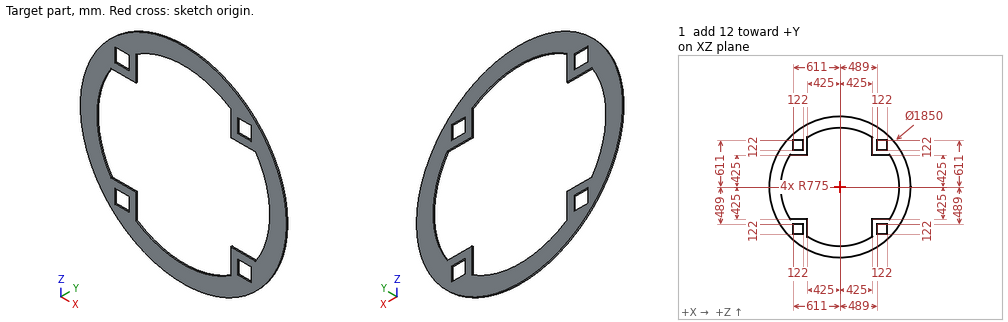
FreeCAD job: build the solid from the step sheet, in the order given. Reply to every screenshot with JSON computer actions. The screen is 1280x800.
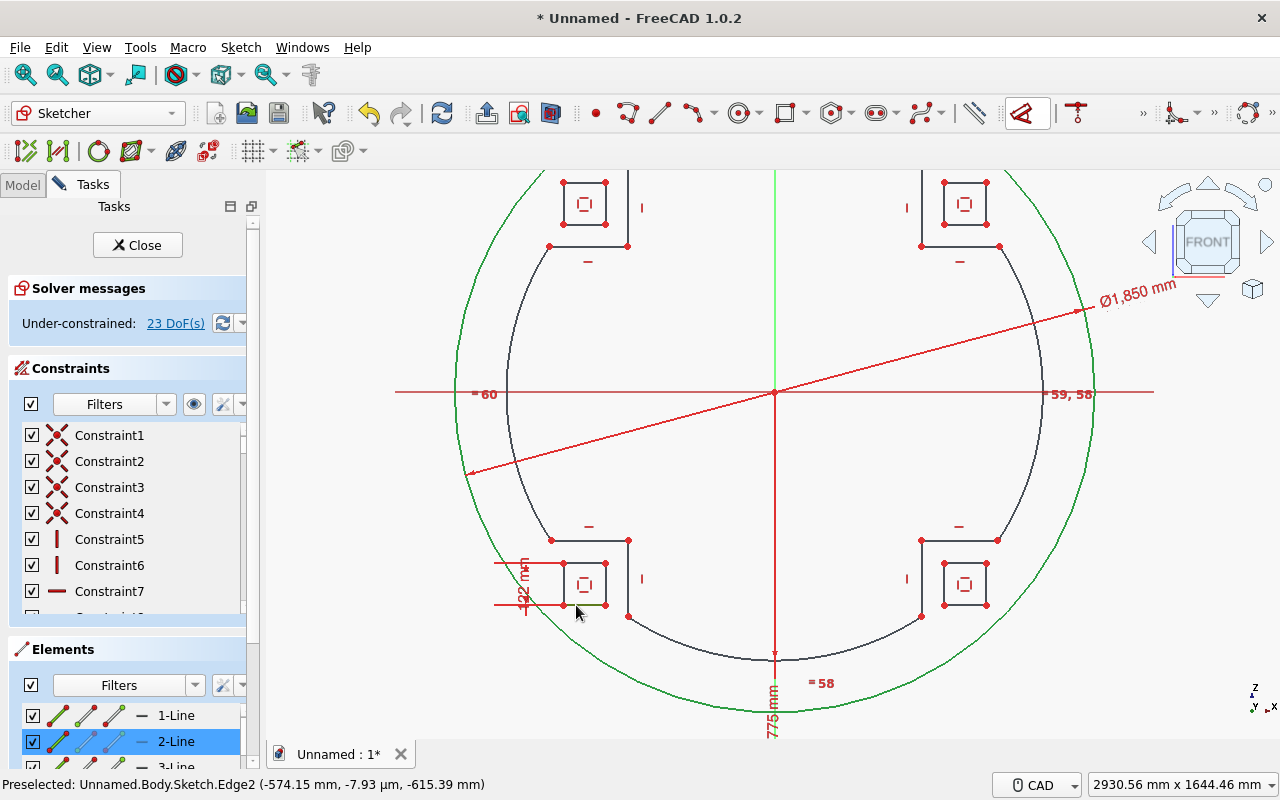
{"action": "key", "text": "l"}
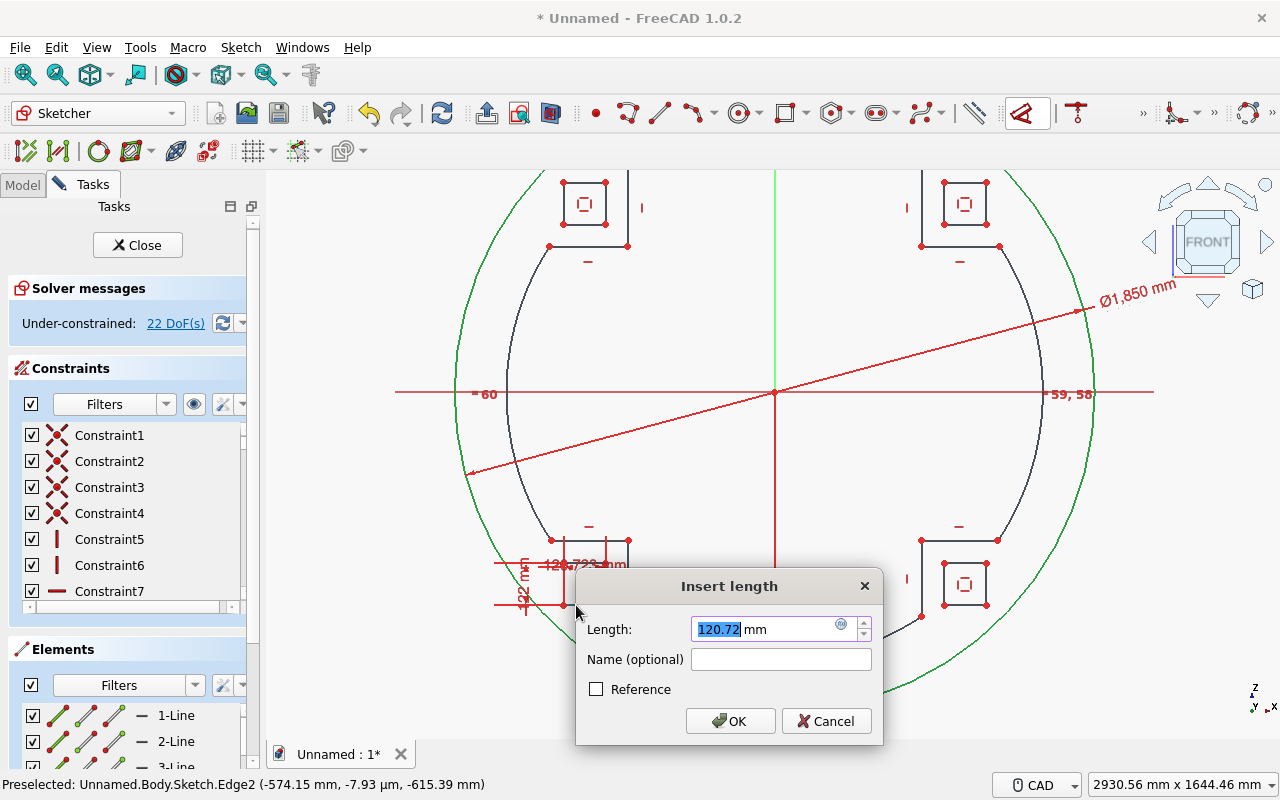
{"action": "type", "text": "122"}
{"action": "key", "text": "Return"}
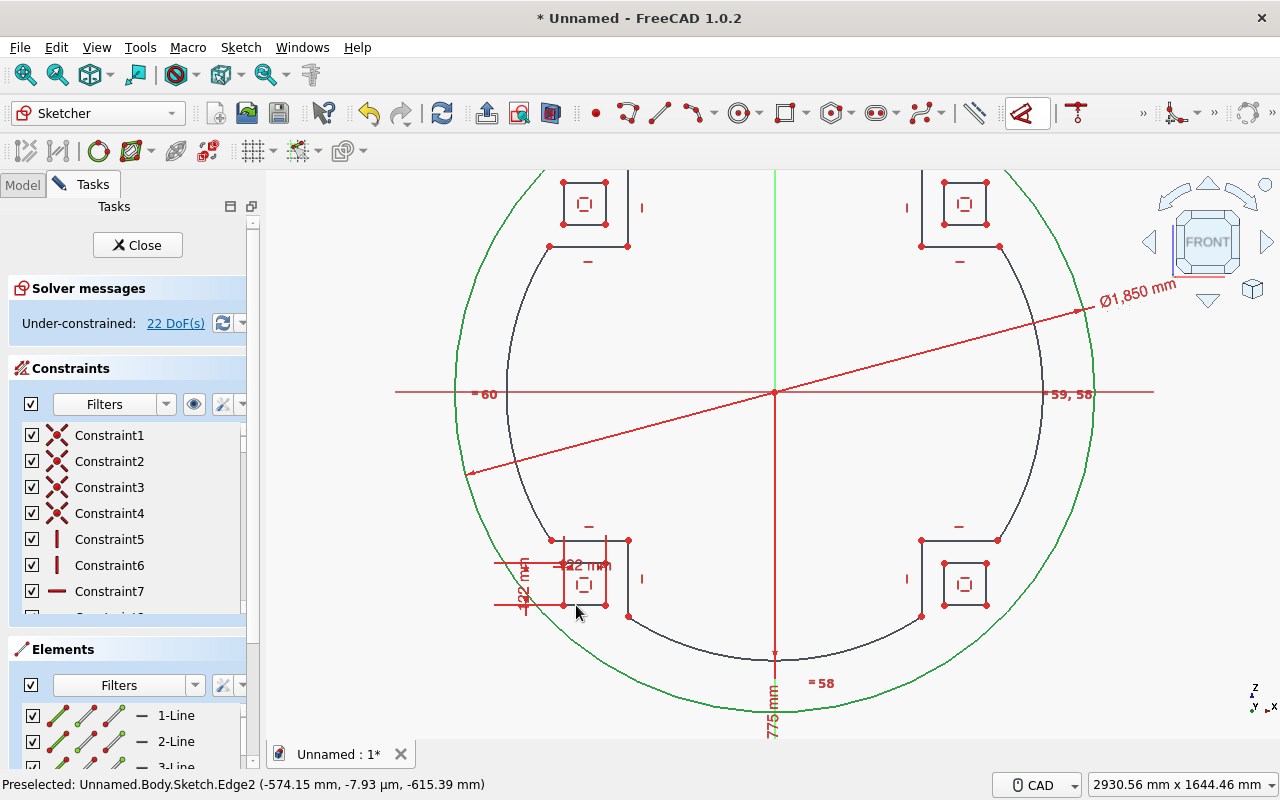
{"action": "left_click", "coordinate": [564, 212]}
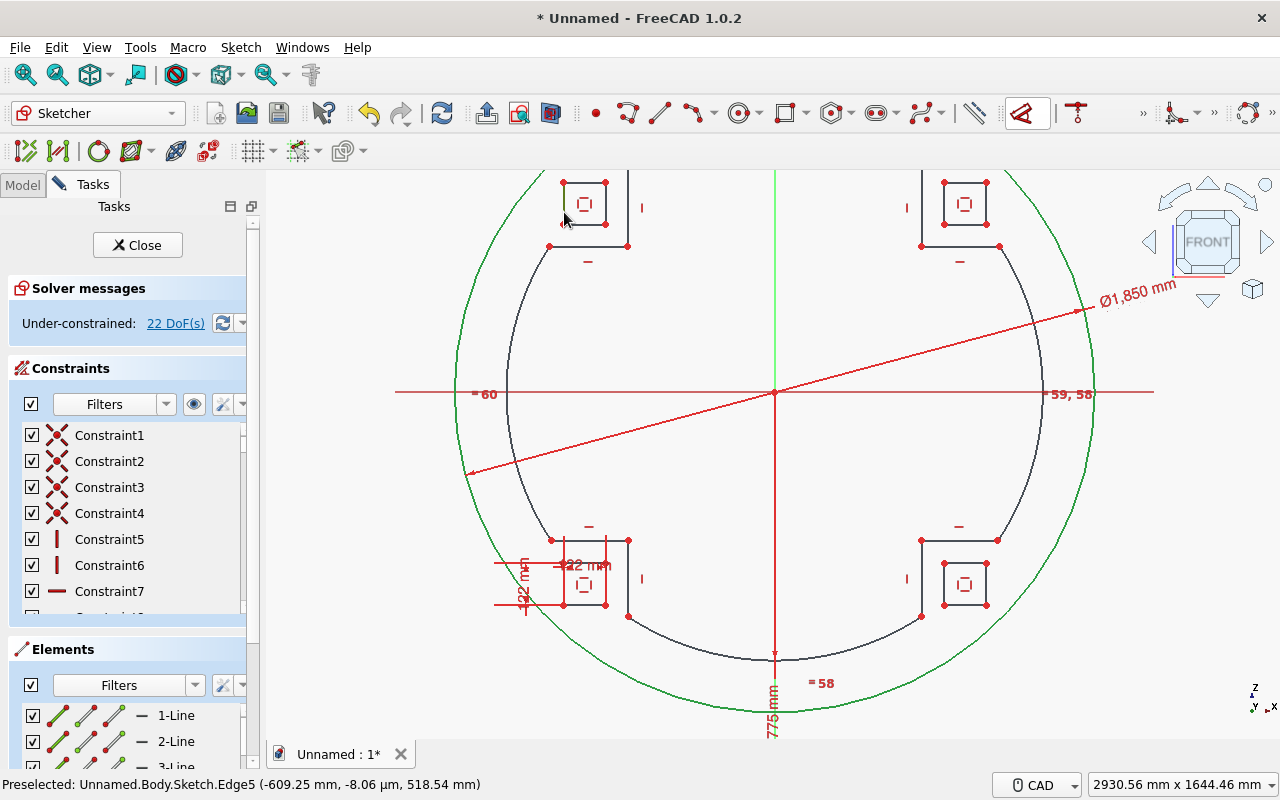
{"action": "key", "text": "i"}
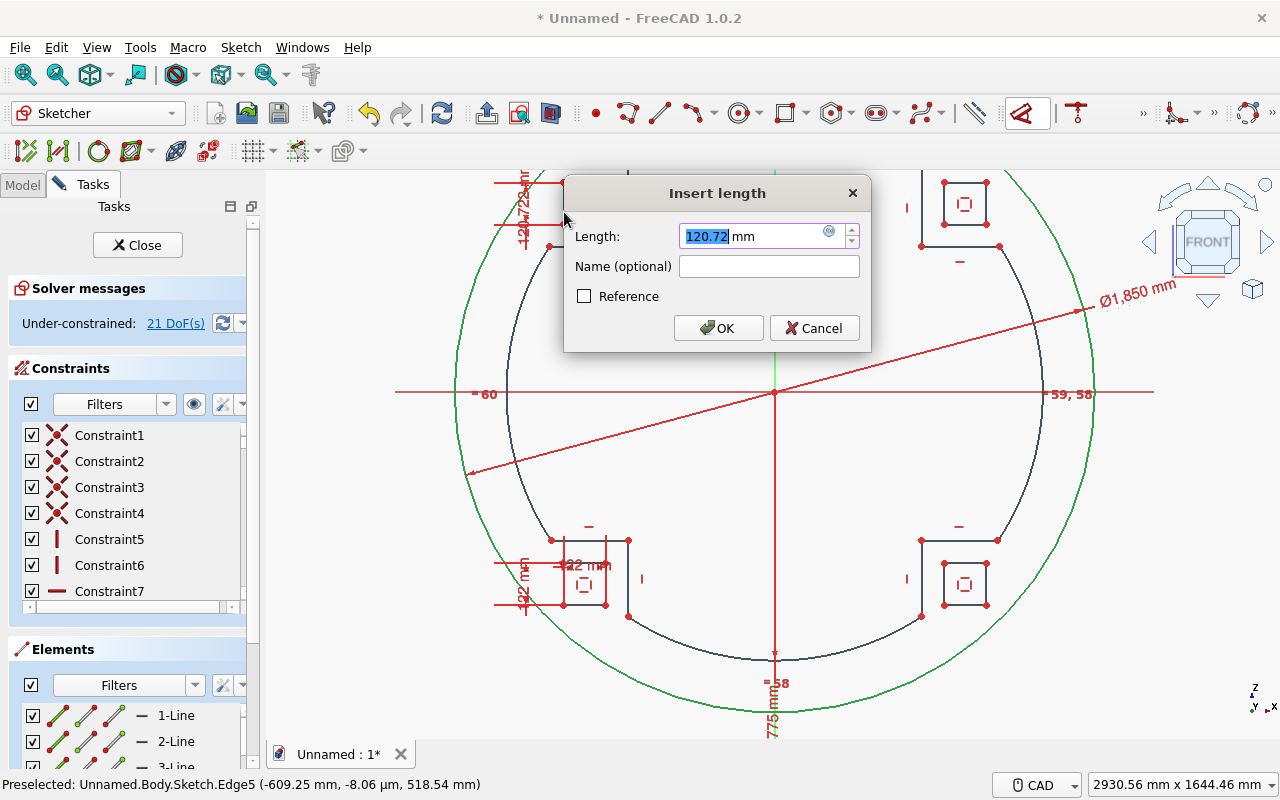
{"action": "type", "text": "122"}
{"action": "key", "text": "Return"}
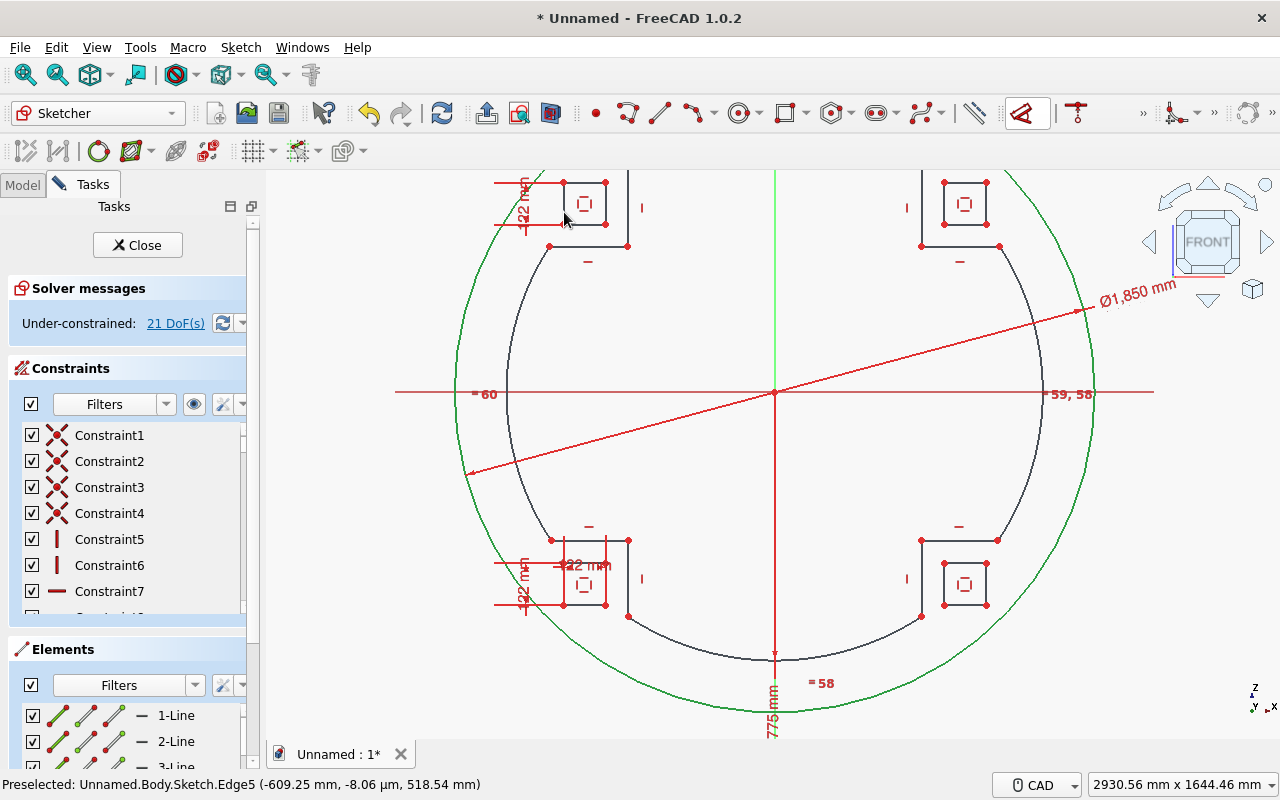
{"action": "left_click", "coordinate": [576, 225]}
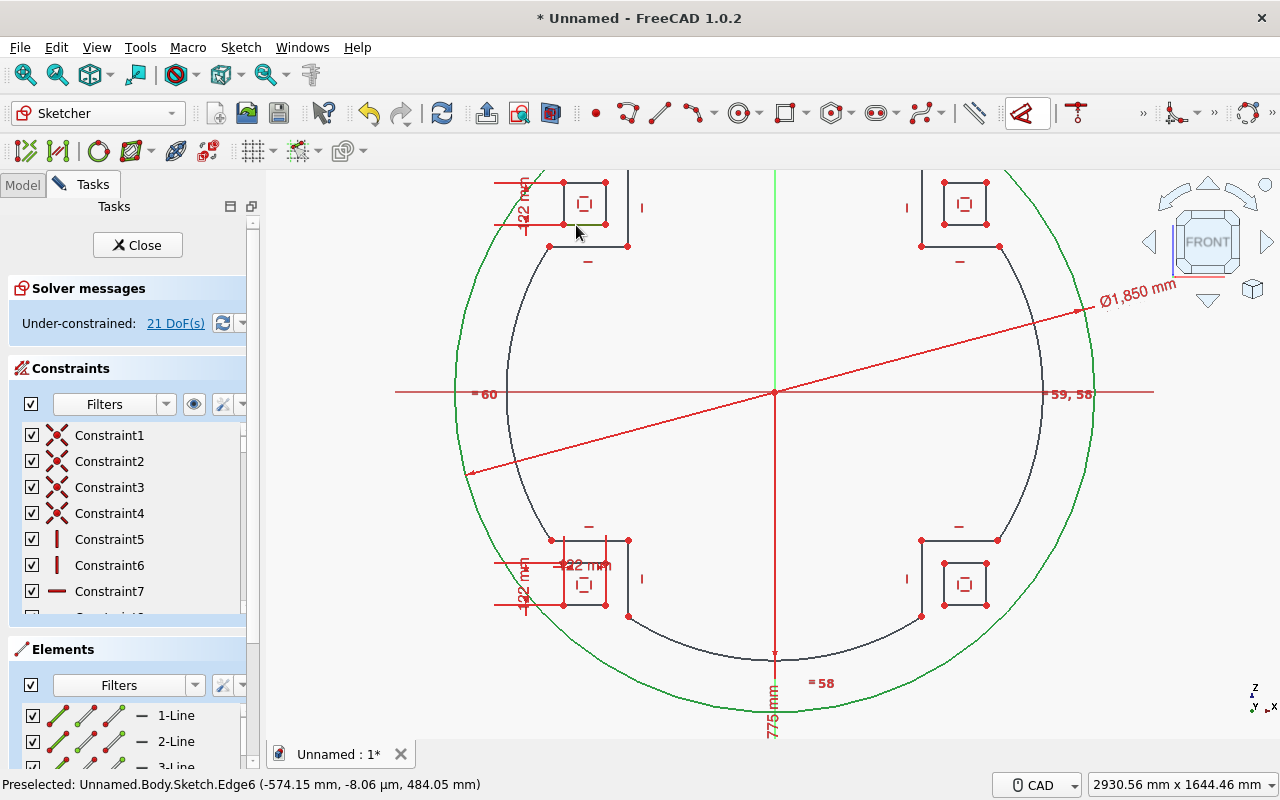
{"action": "key", "text": "l"}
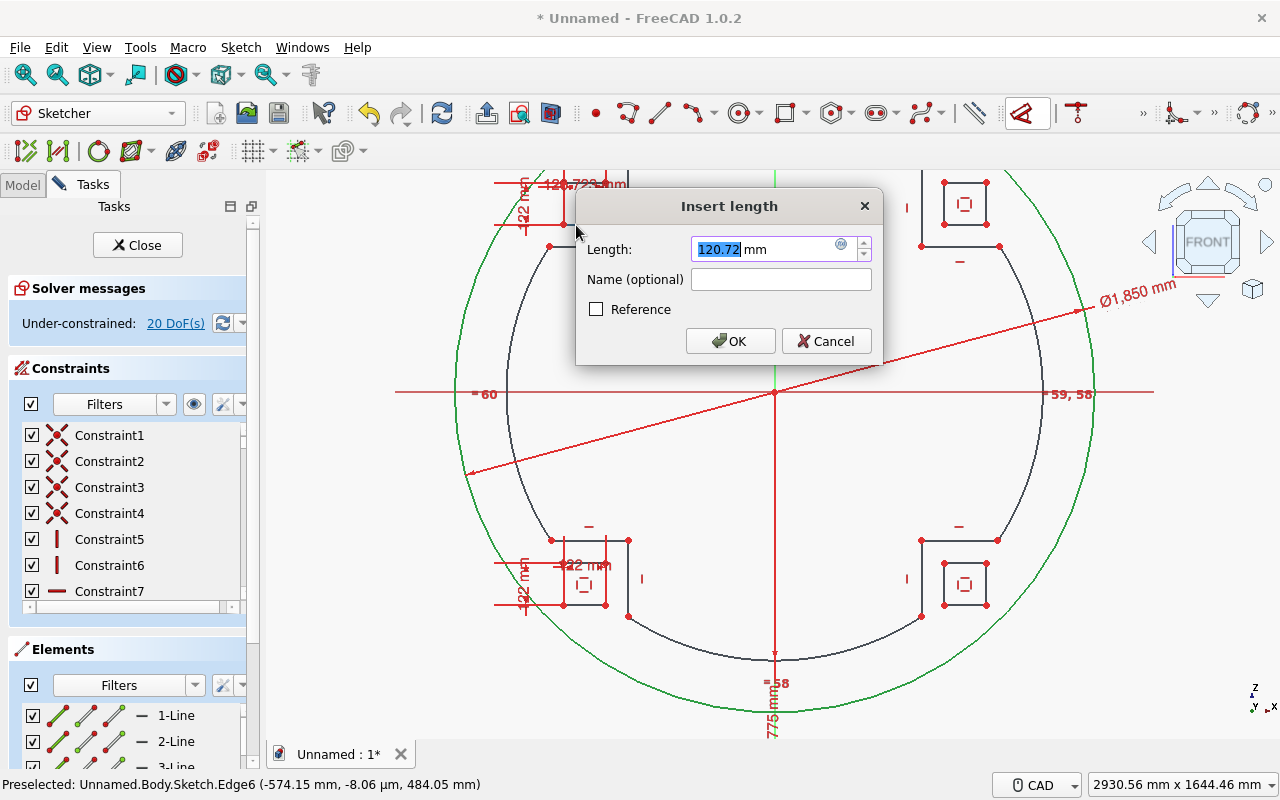
{"action": "type", "text": "122"}
{"action": "key", "text": "Return"}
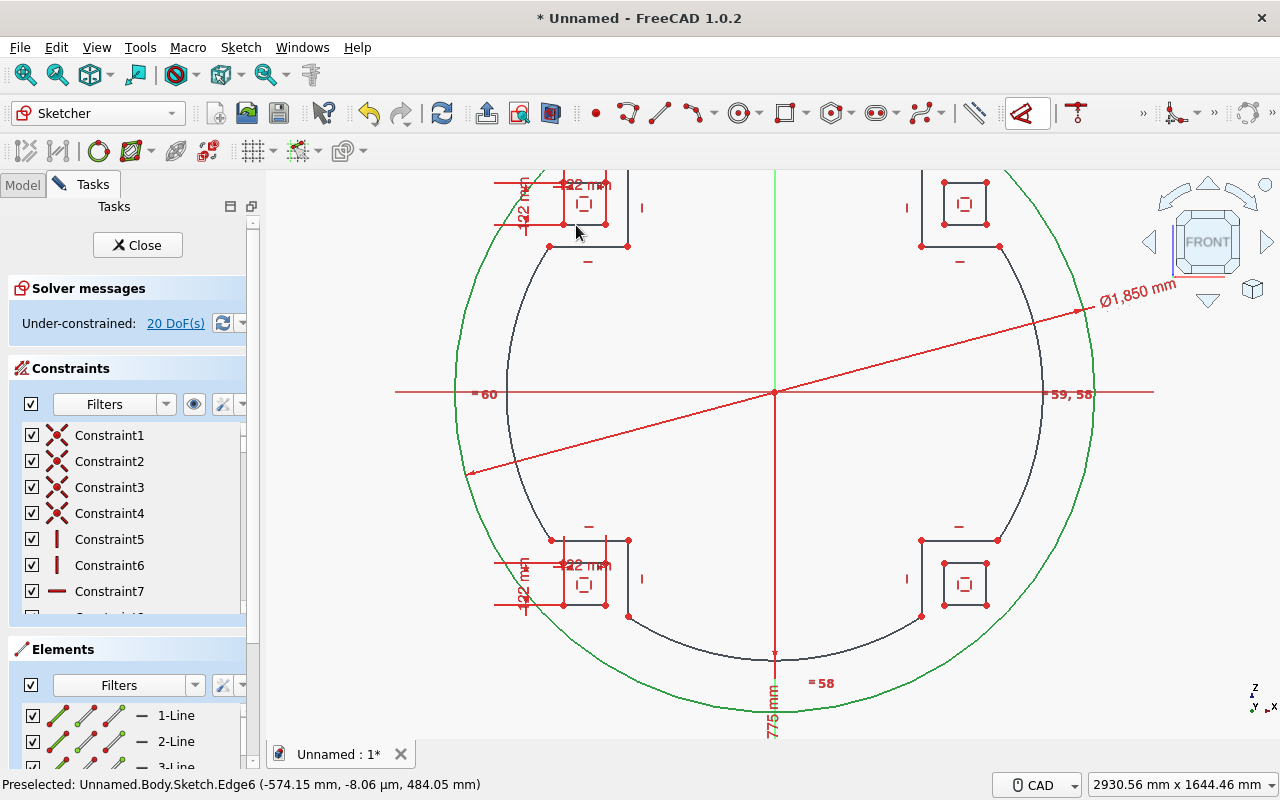
{"action": "left_click", "coordinate": [944, 576]}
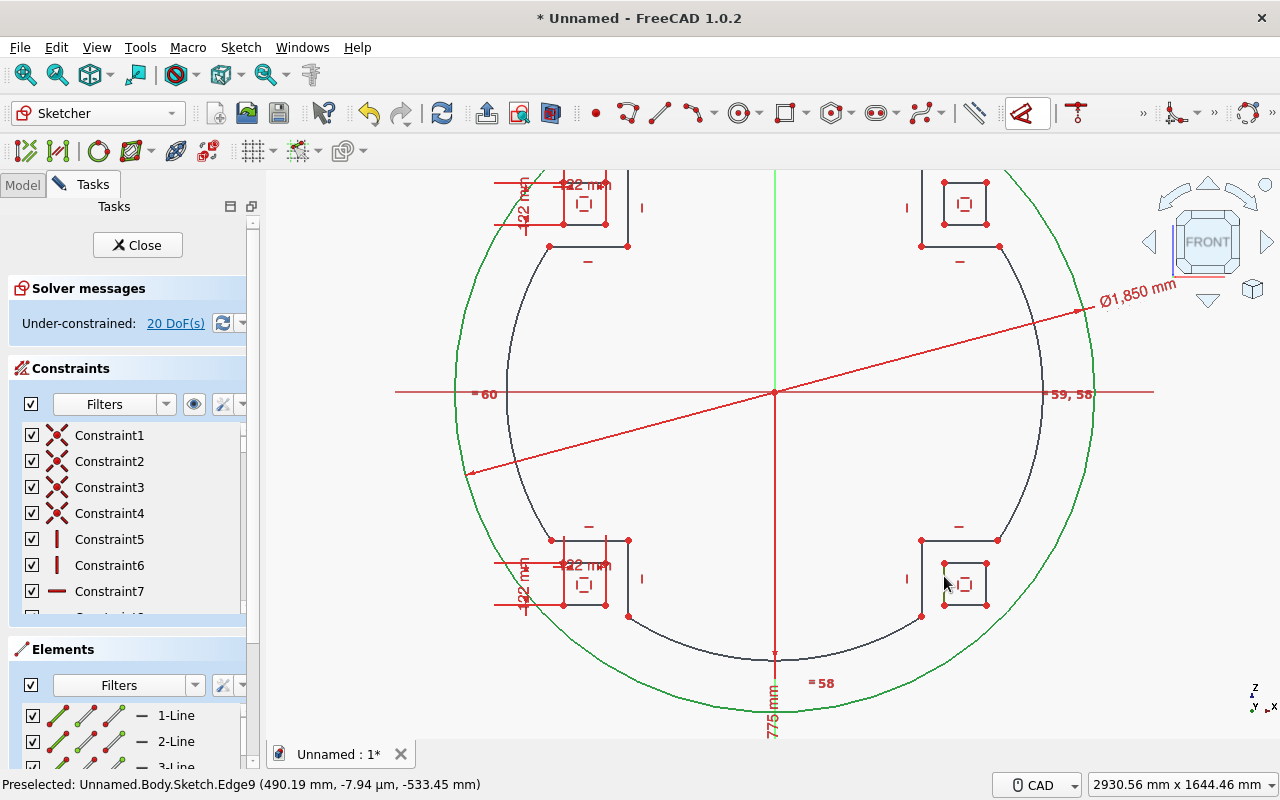
{"action": "key", "text": "i"}